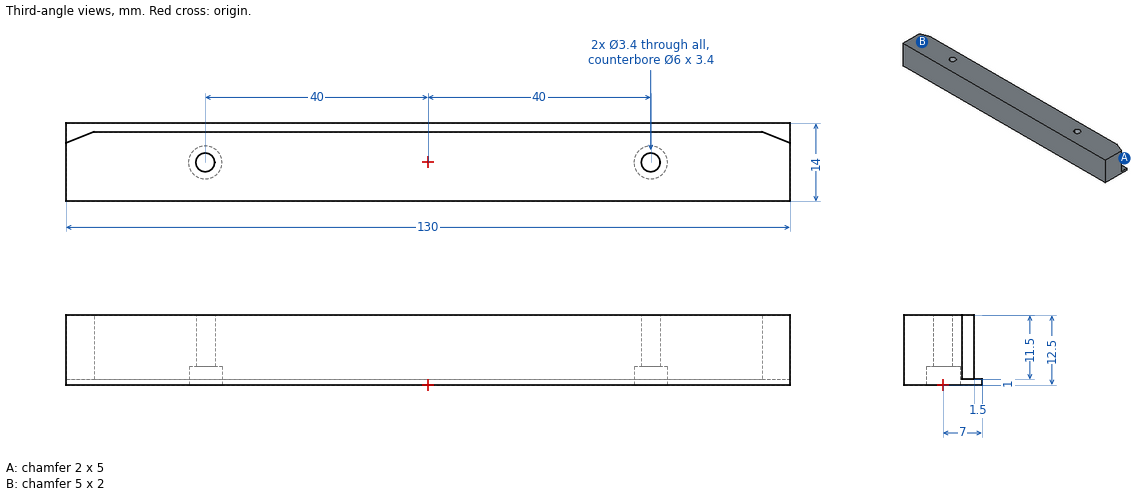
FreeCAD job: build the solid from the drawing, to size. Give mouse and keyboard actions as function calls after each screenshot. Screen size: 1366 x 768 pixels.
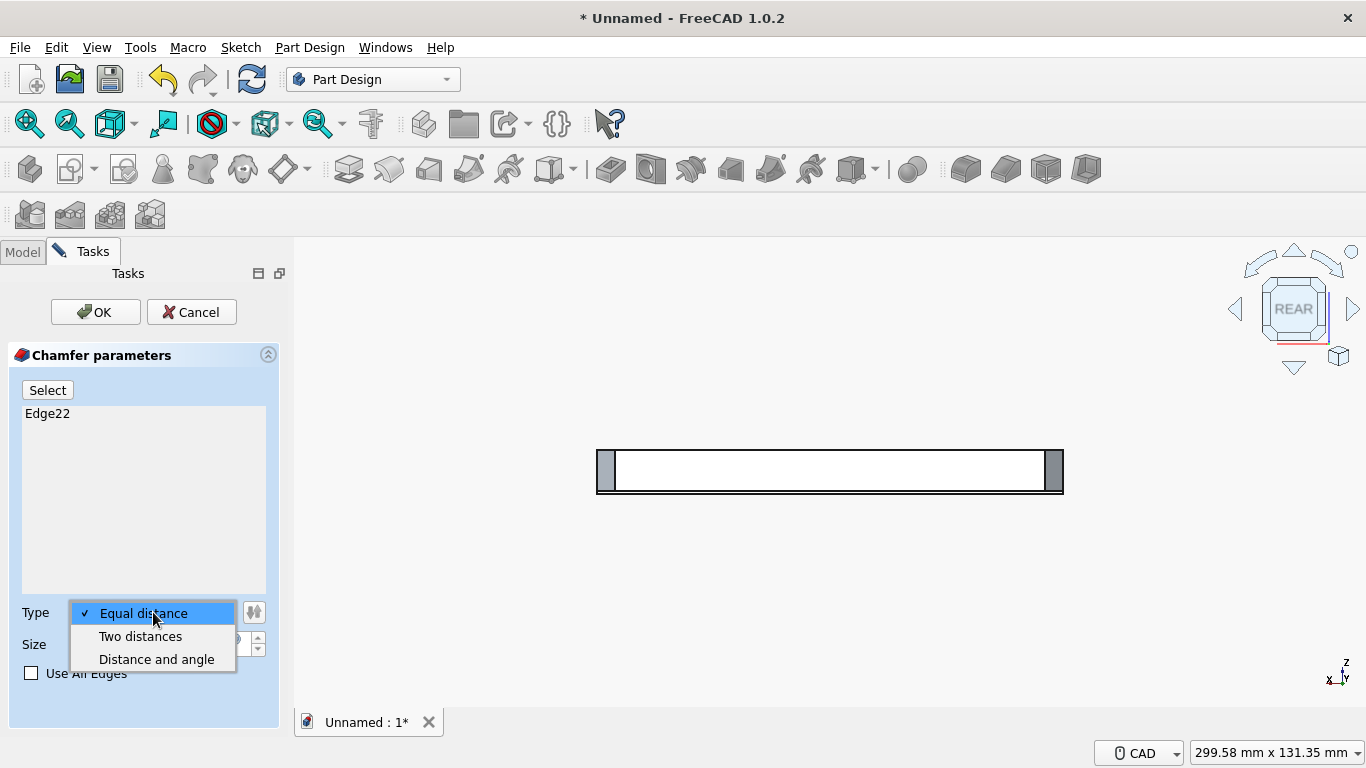
click(152, 636)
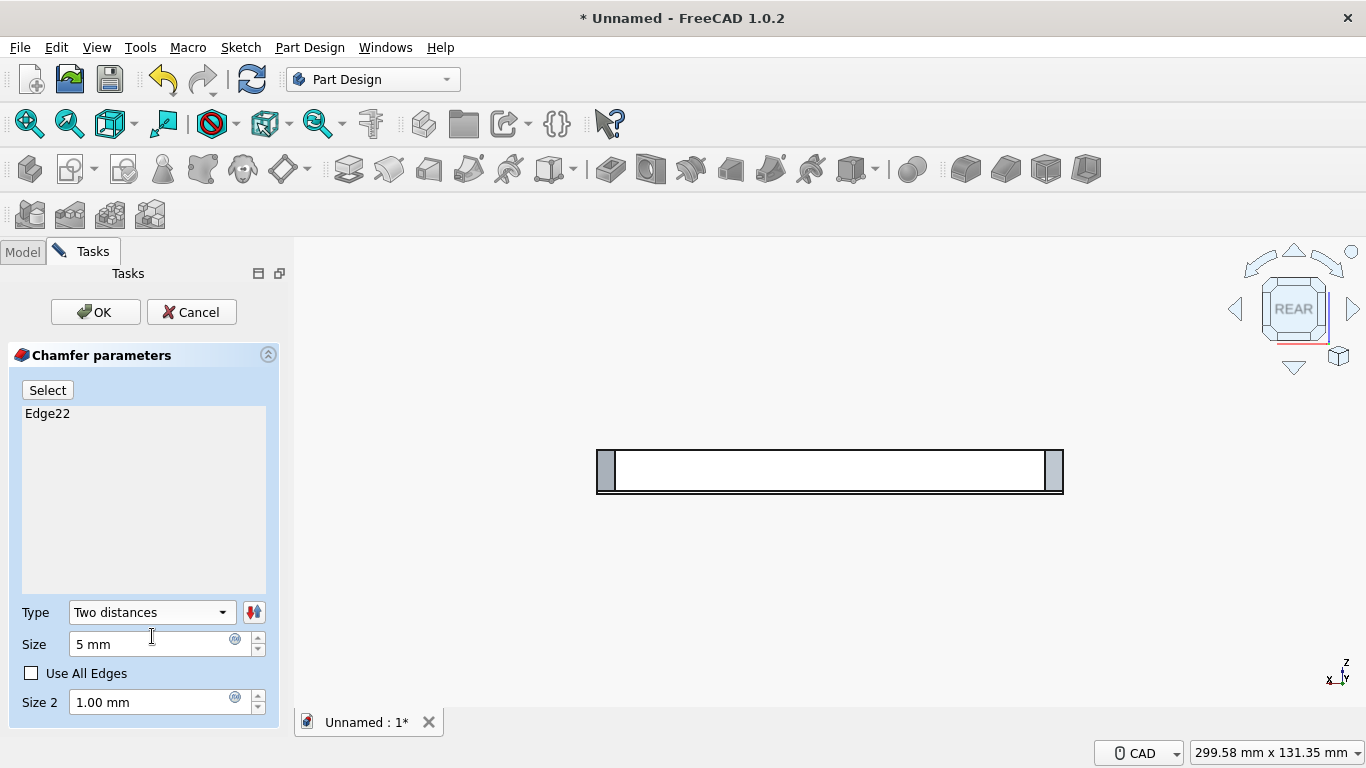
triple_click(160, 702)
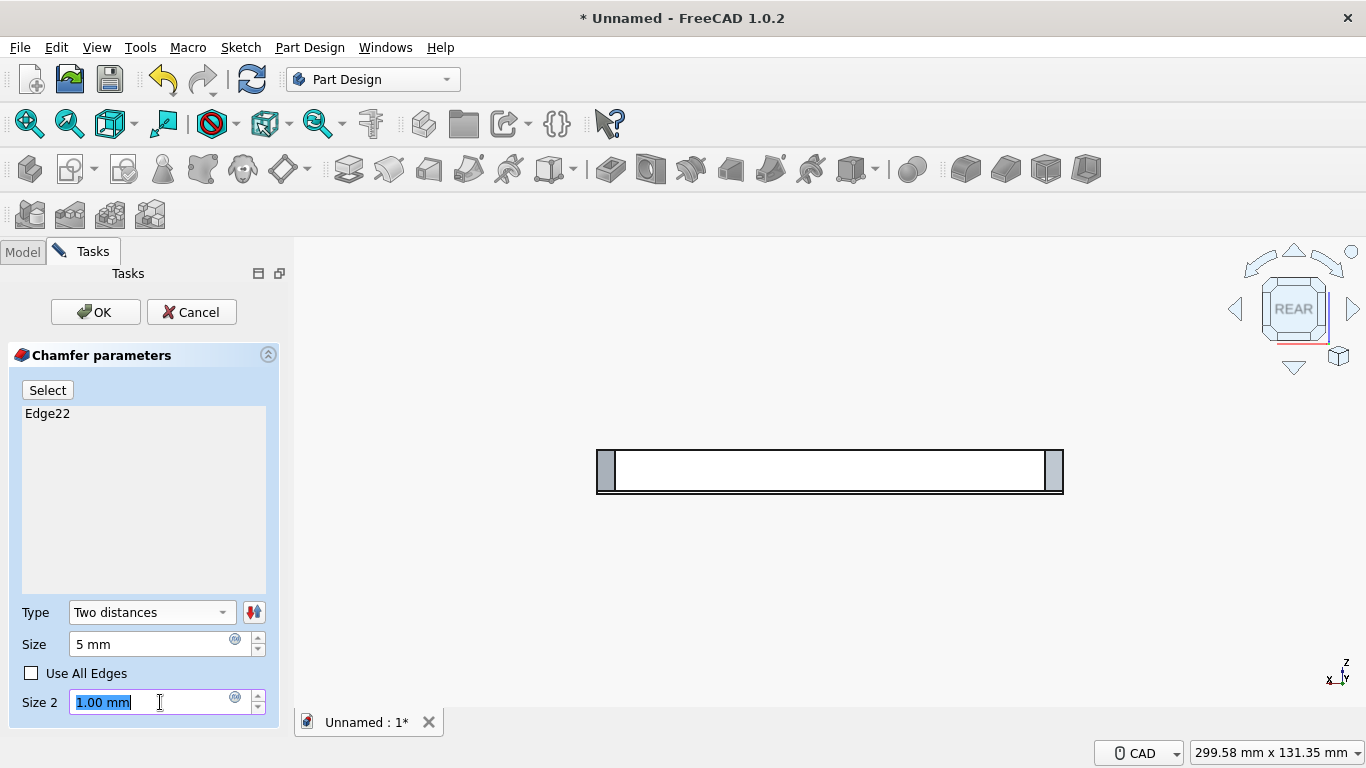
text(2)
key(Tab)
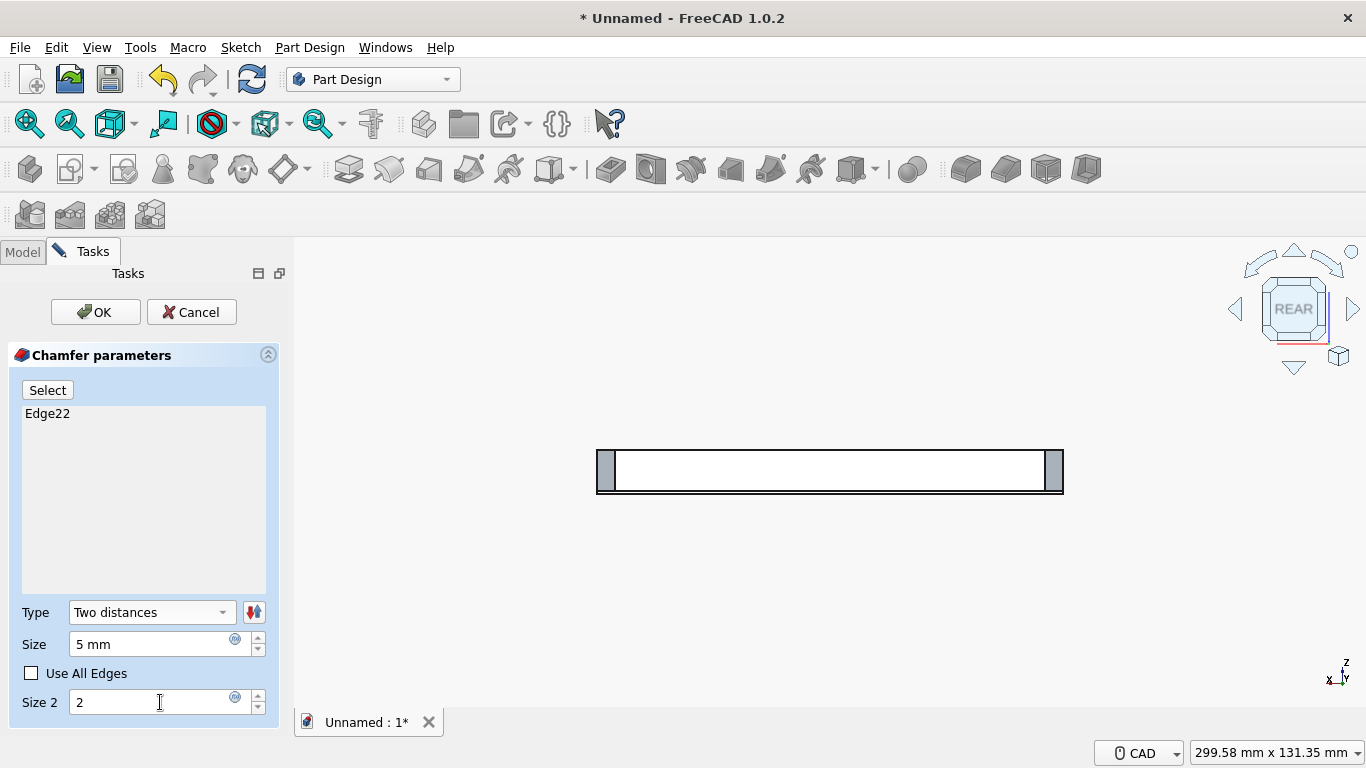
click(96, 312)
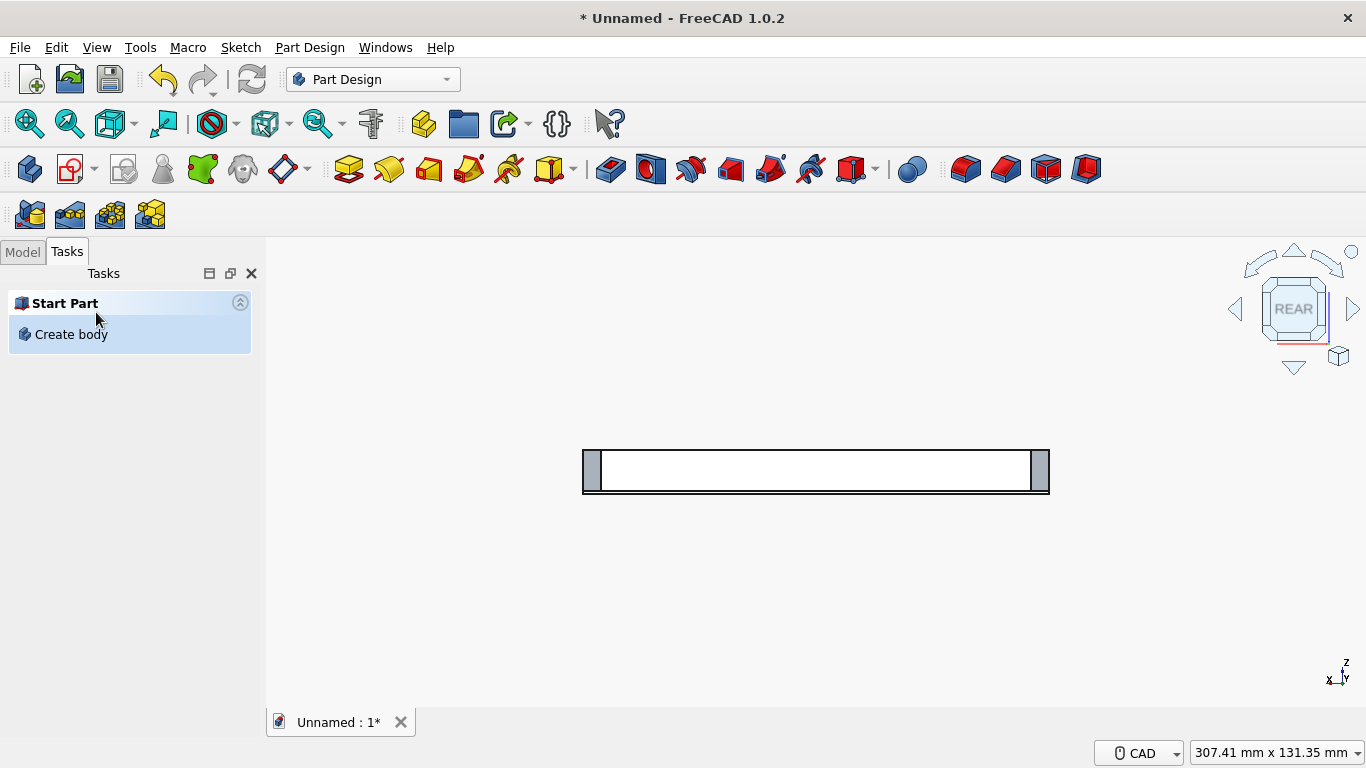
click(30, 124)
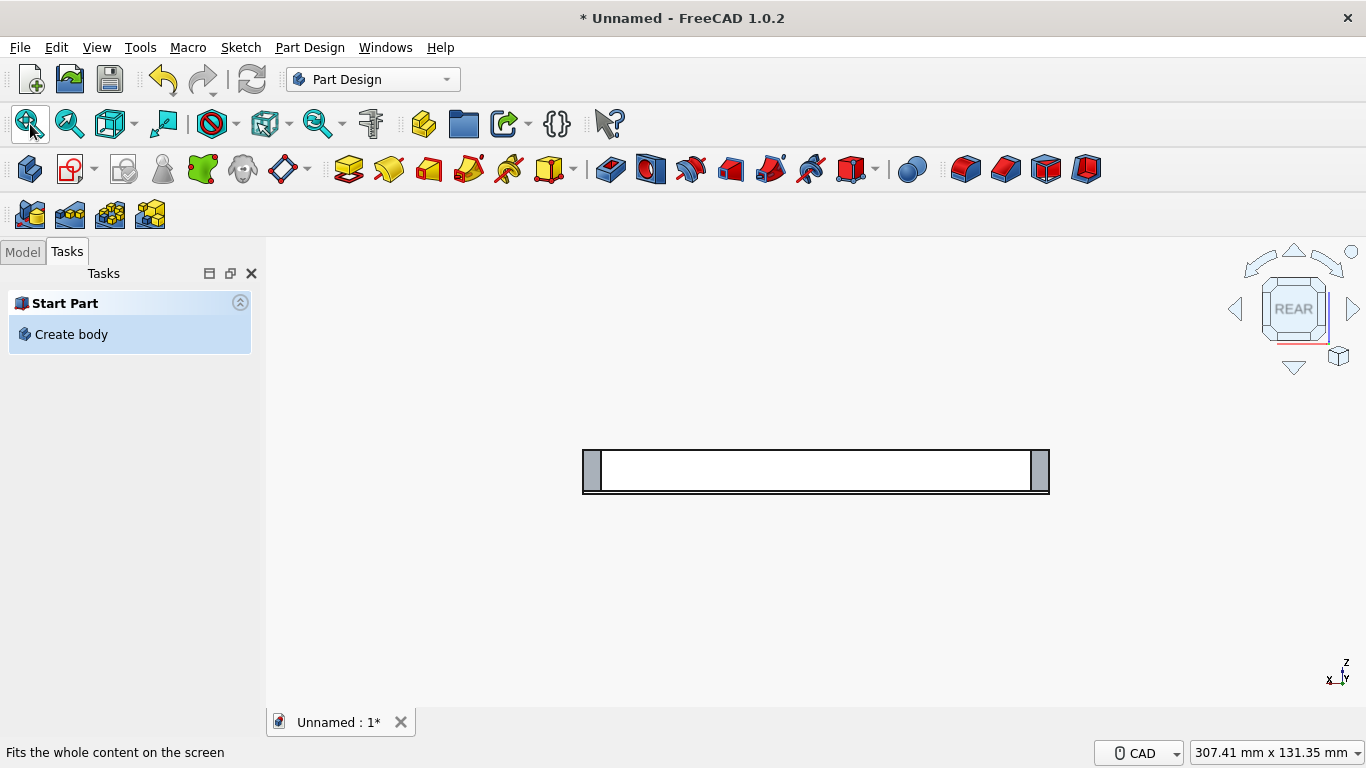
key(5)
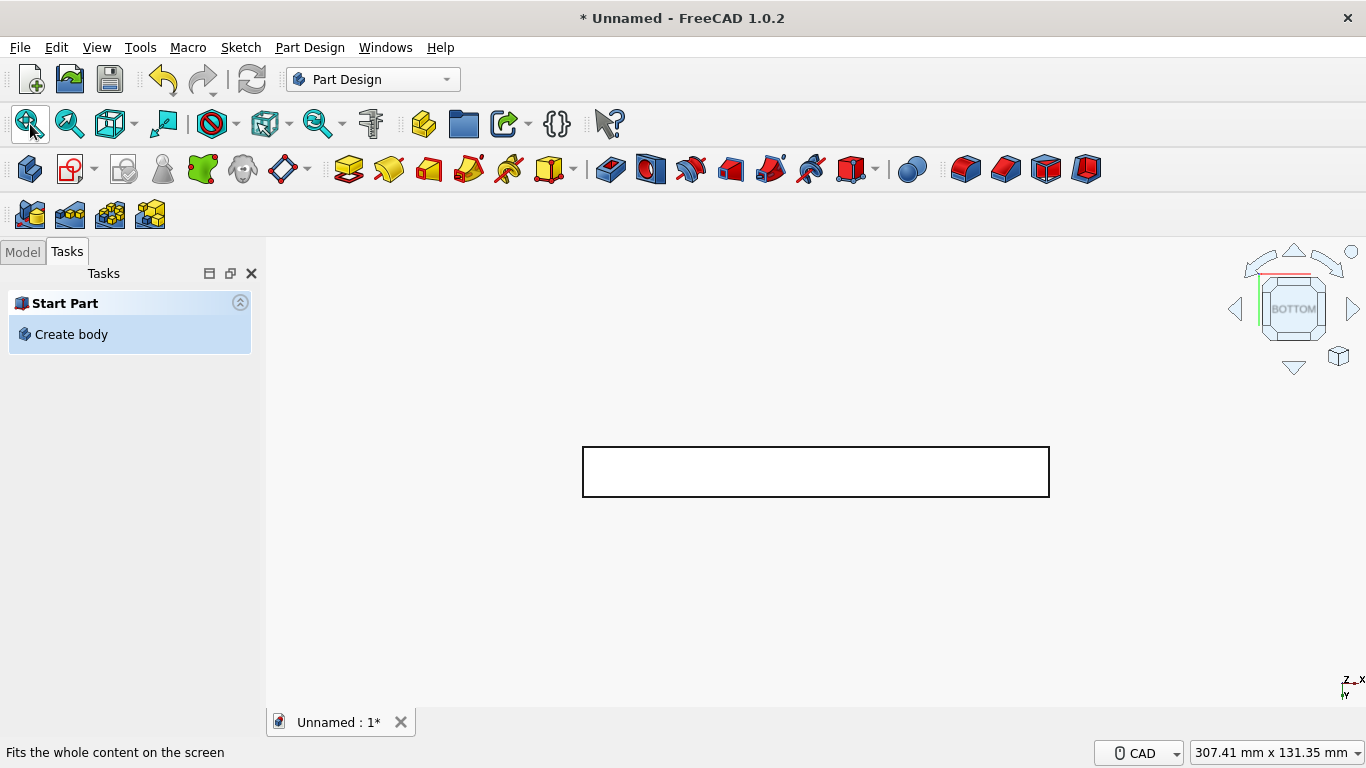
click(30, 124)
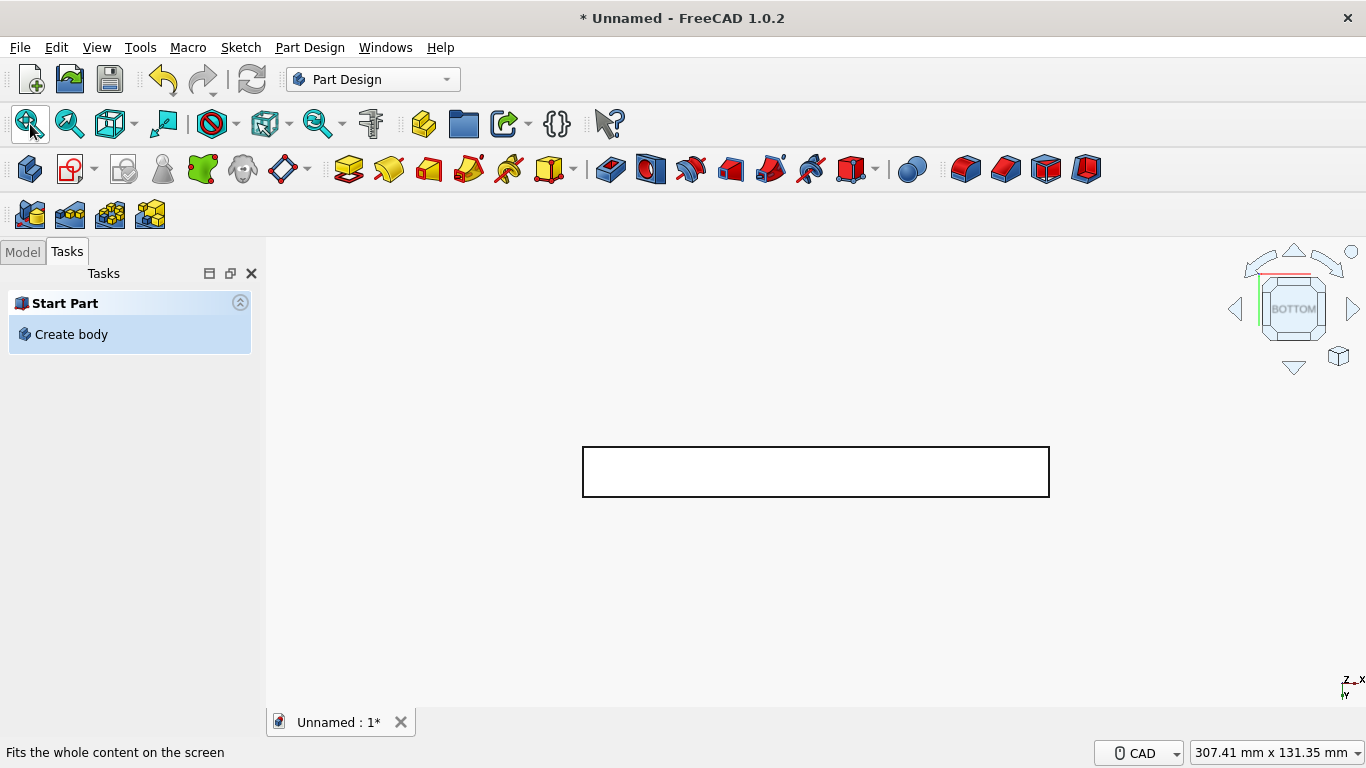
click(1015, 471)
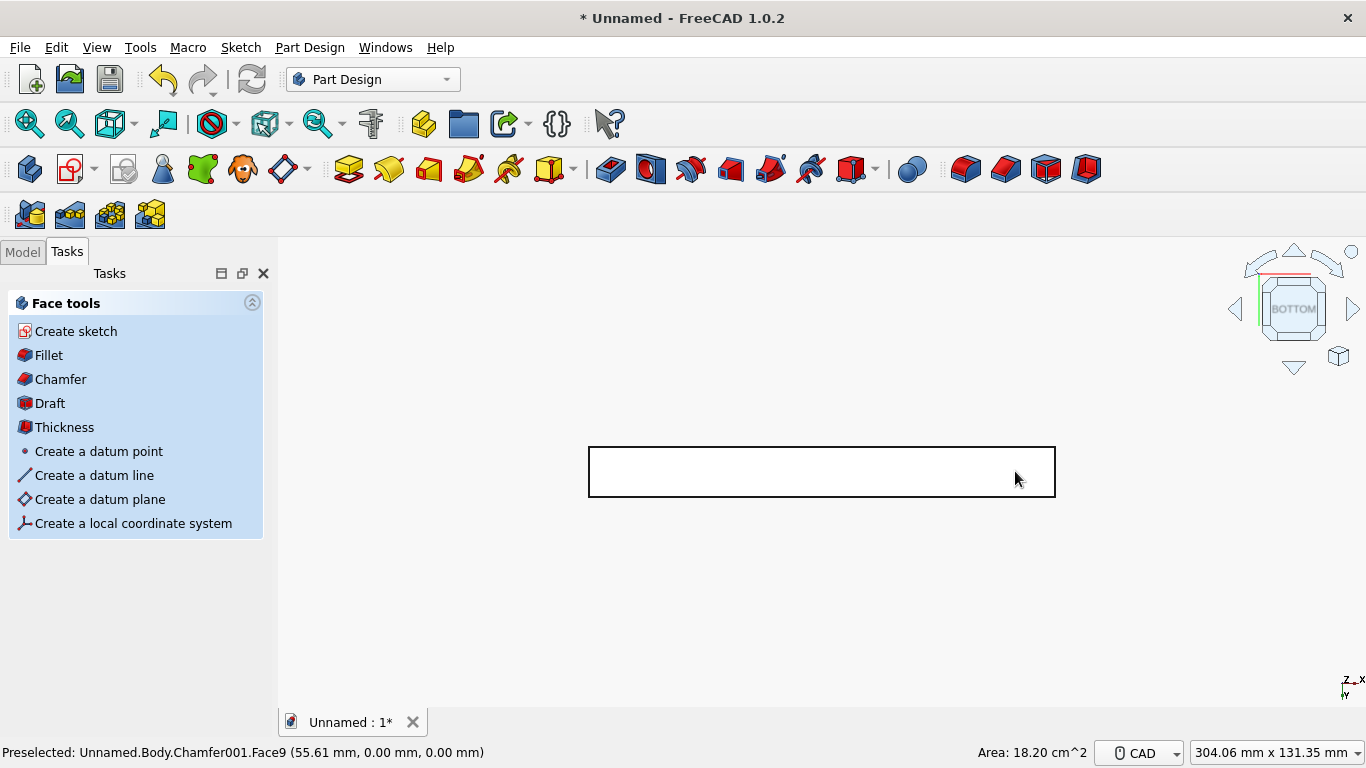
click(70, 170)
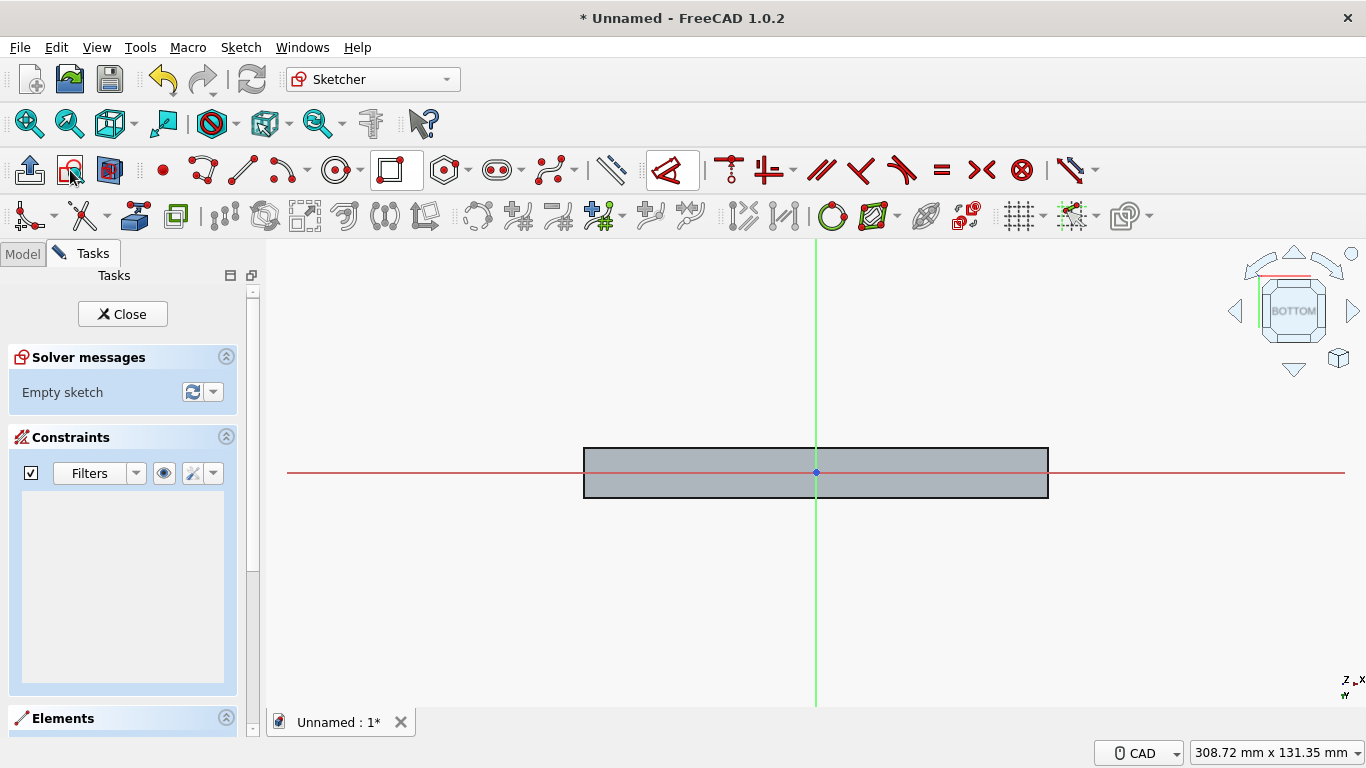
scroll(872, 473, up, 4)